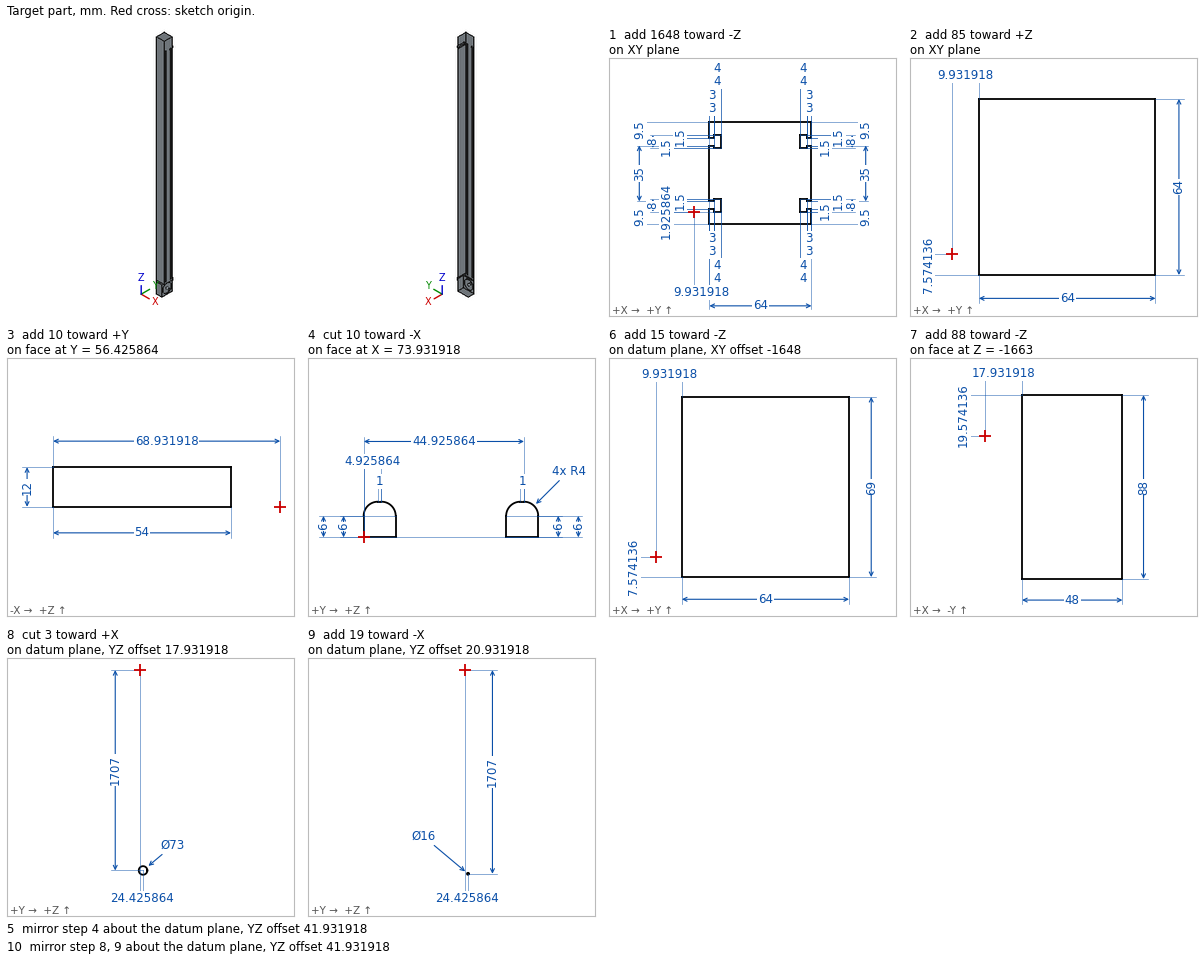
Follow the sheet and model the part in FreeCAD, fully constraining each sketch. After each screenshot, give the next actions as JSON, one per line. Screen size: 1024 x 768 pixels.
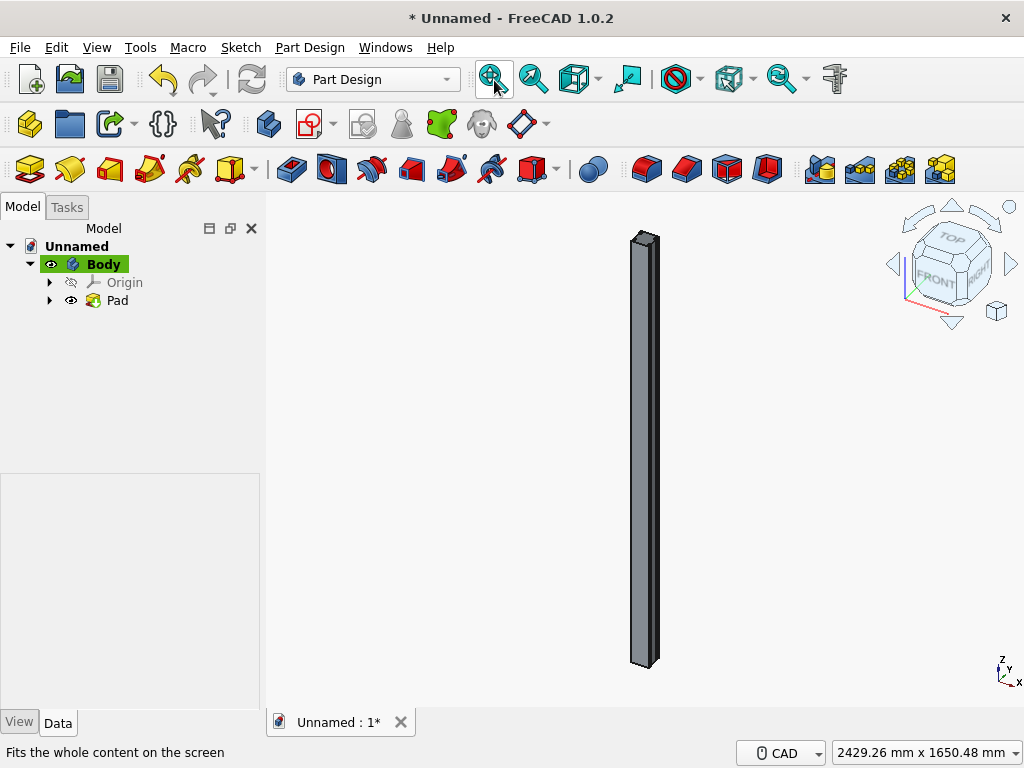
{"action": "left_click", "coordinate": [310, 124]}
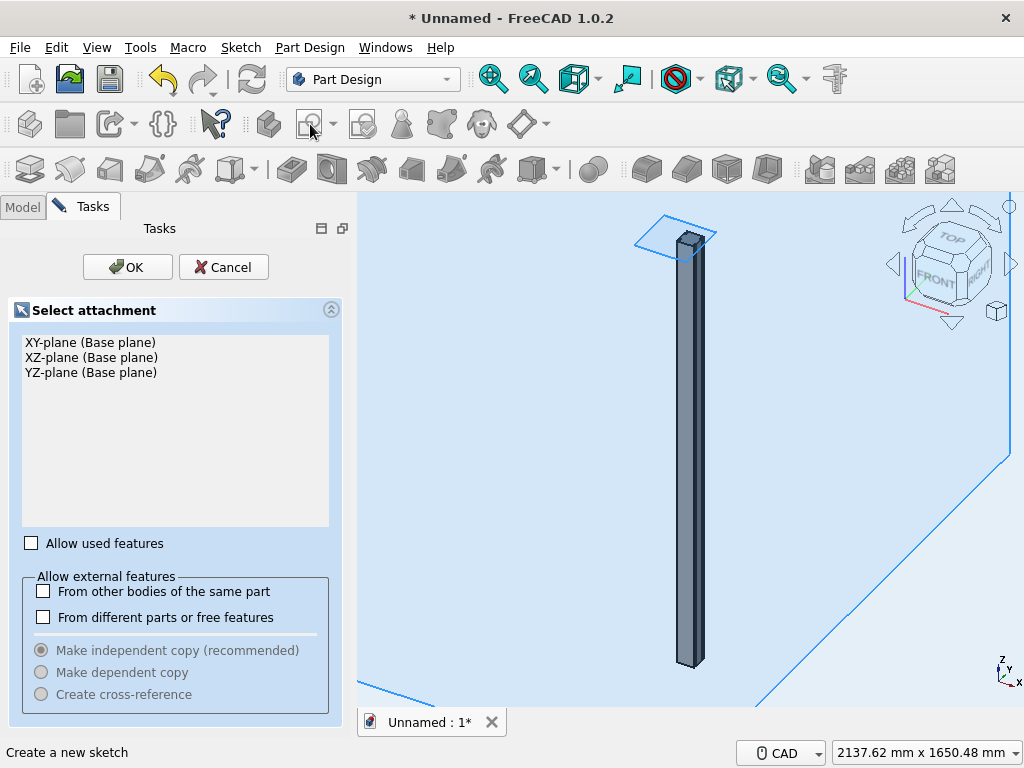
{"action": "left_click", "coordinate": [82, 342]}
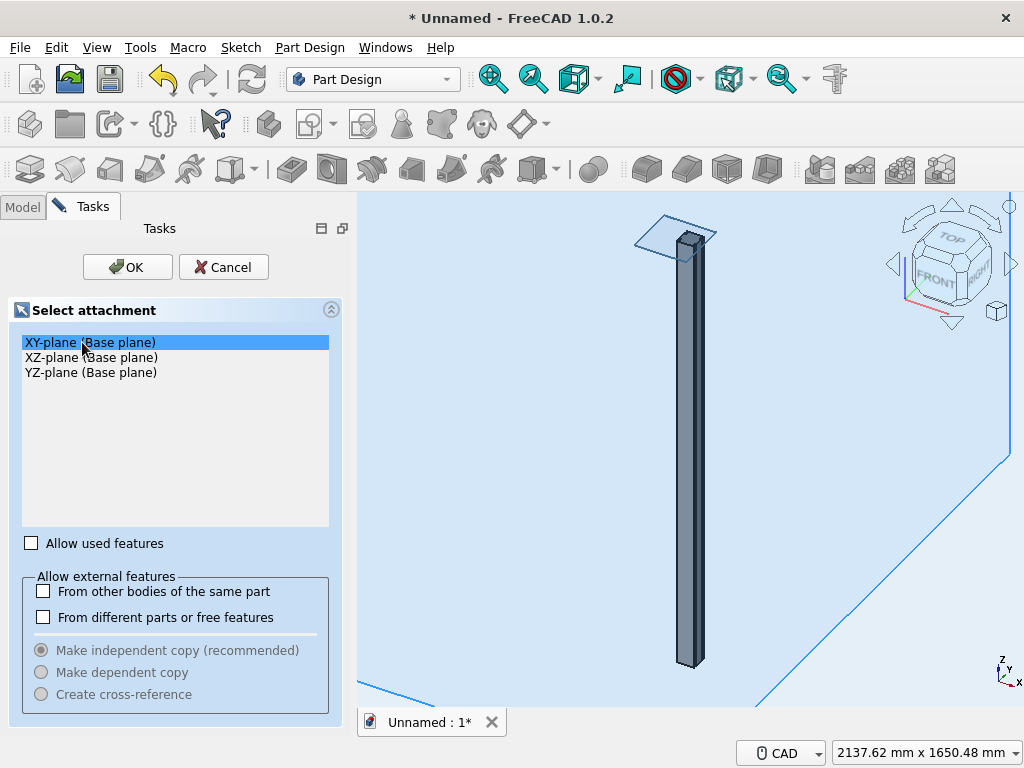
{"action": "left_click", "coordinate": [128, 267]}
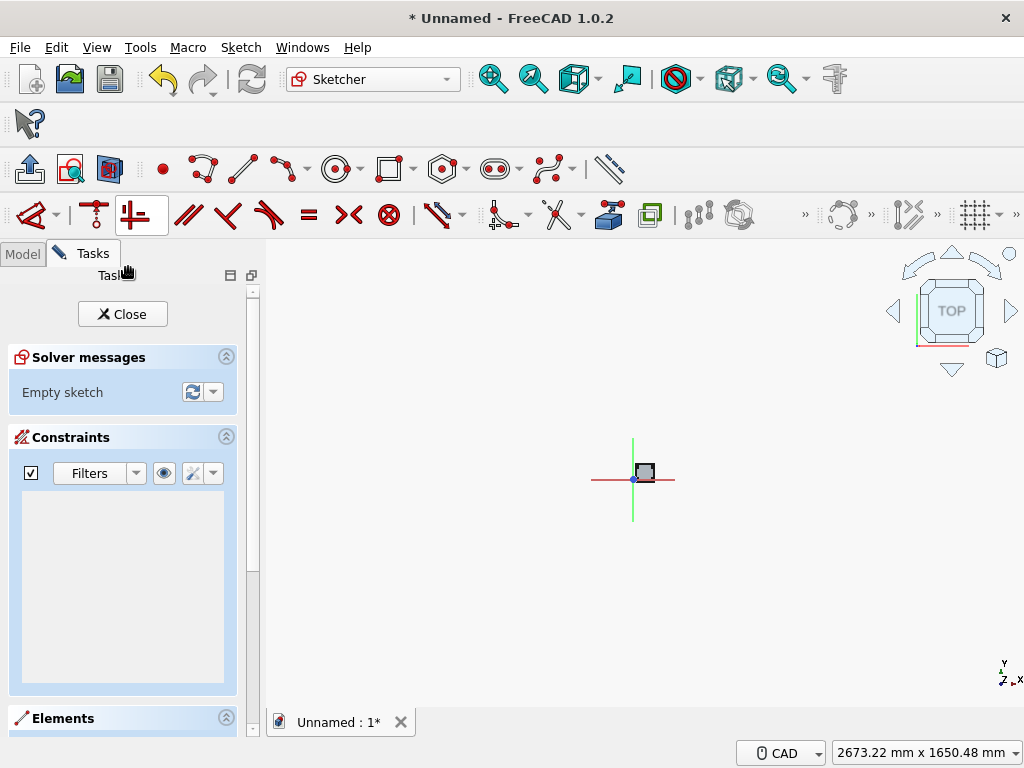
{"action": "scroll", "coordinate": [648, 473], "scroll_direction": "up", "scroll_amount": 14}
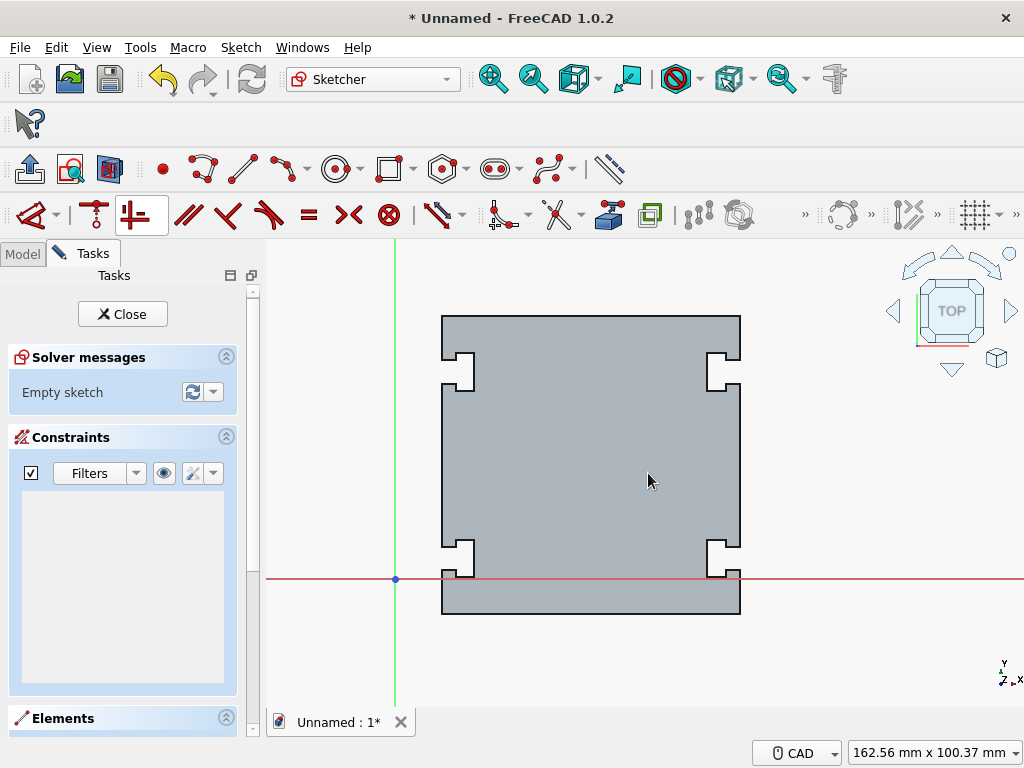
{"action": "left_click", "coordinate": [390, 170]}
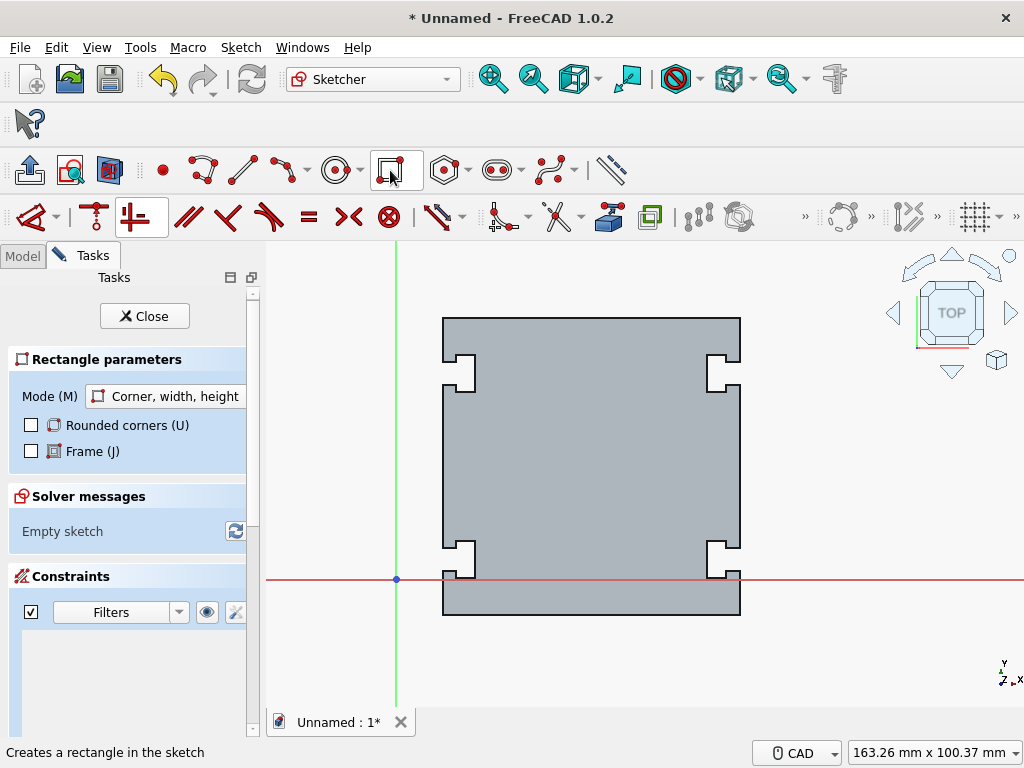
{"action": "left_click", "coordinate": [443, 318]}
{"action": "mouse_move", "coordinate": [740, 615]}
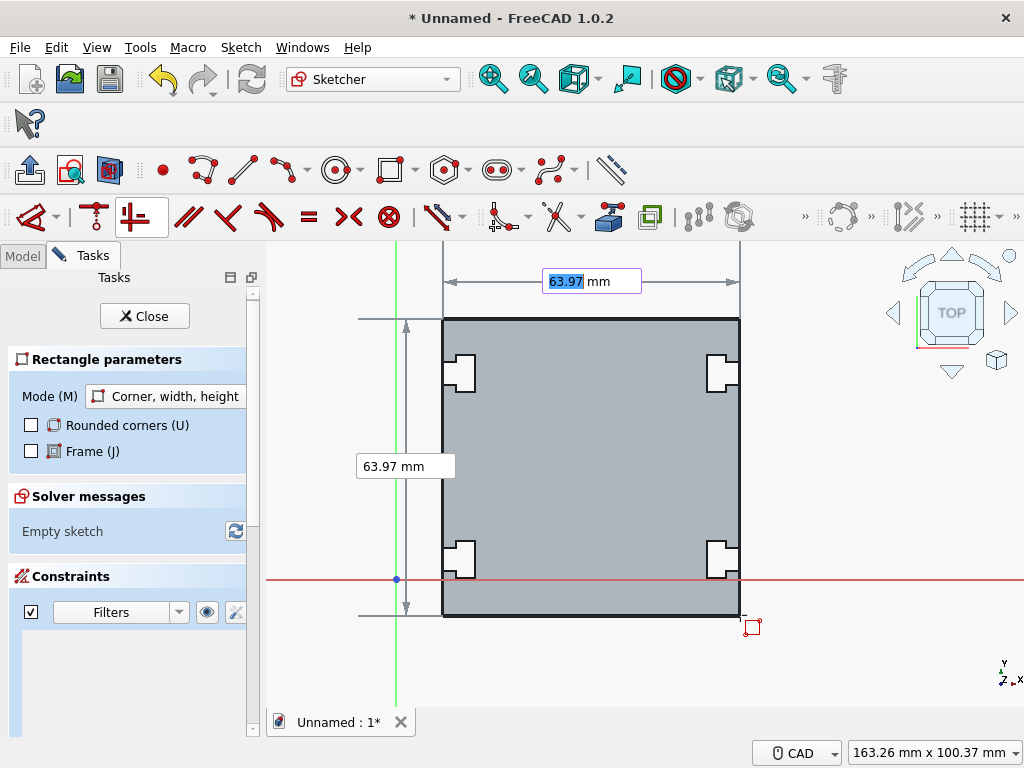
{"action": "type", "text": "64"}
{"action": "key", "text": "Tab"}
{"action": "type", "text": "64"}
{"action": "key", "text": "Return"}
{"action": "key", "text": "Escape"}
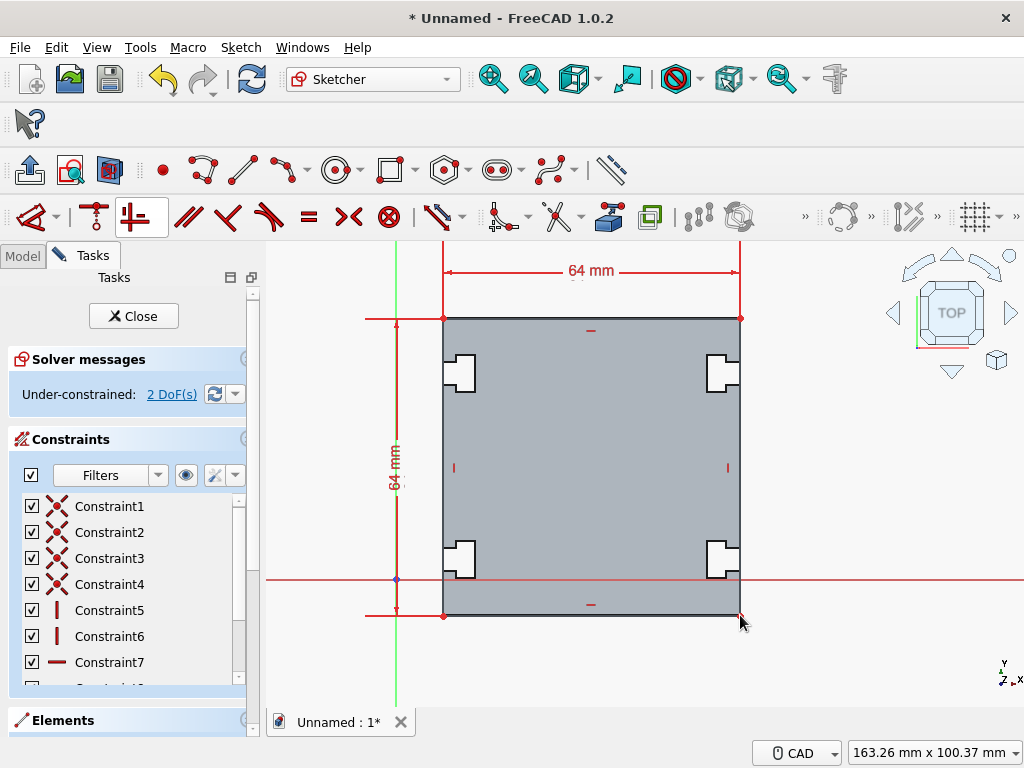
{"action": "left_click", "coordinate": [32, 218]}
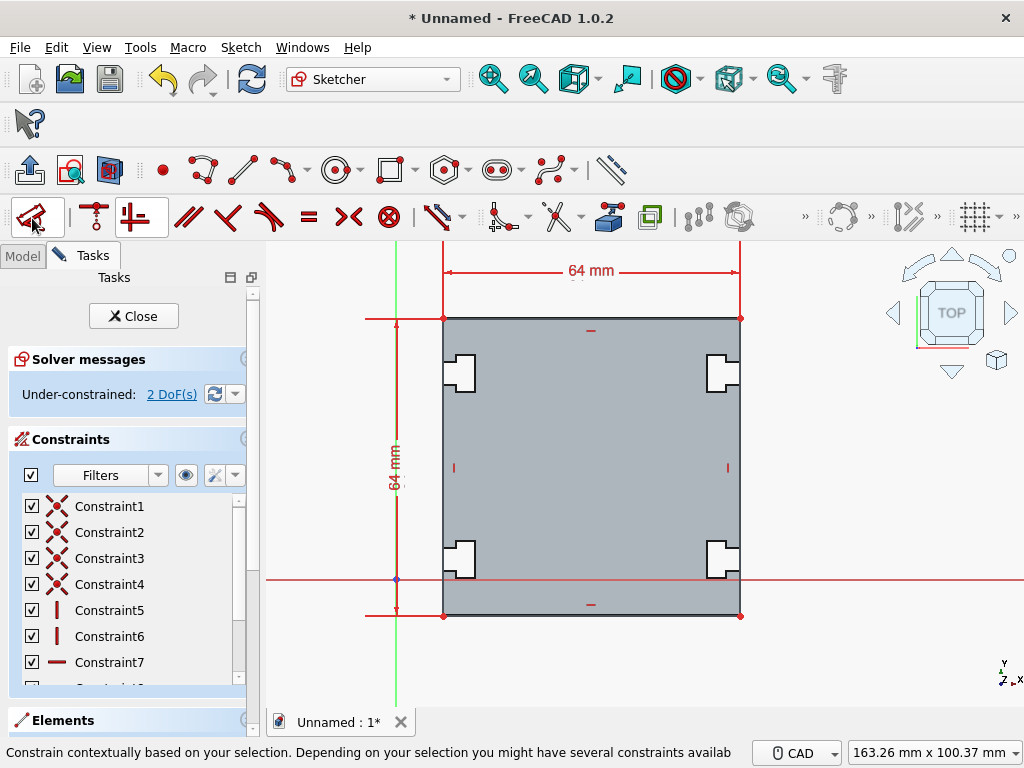
{"action": "left_click", "coordinate": [443, 319]}
{"action": "left_click", "coordinate": [420, 285]}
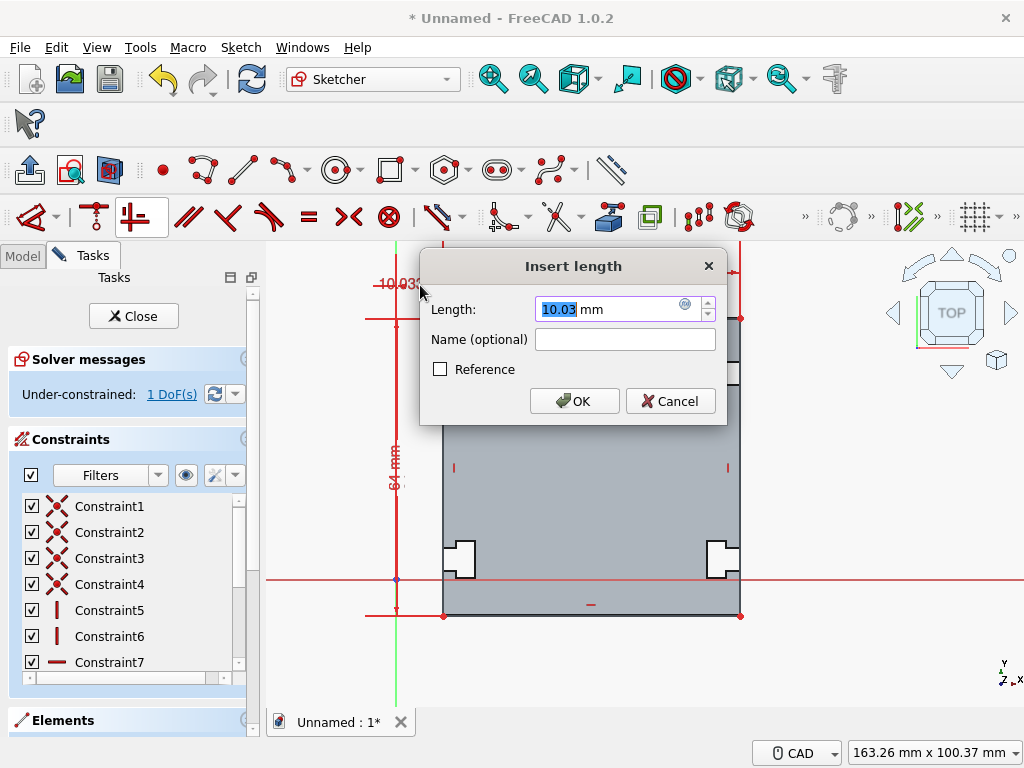
{"action": "type", "text": "9.931918"}
{"action": "key", "text": "Return"}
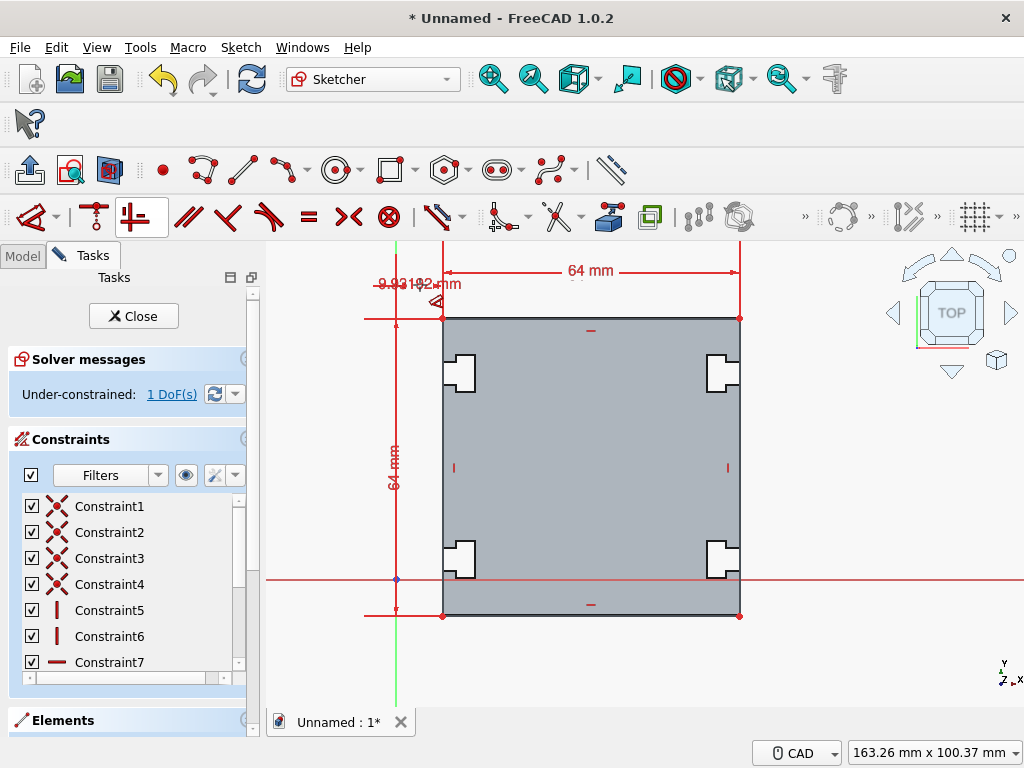
{"action": "left_click", "coordinate": [443, 616]}
{"action": "left_click", "coordinate": [362, 598]}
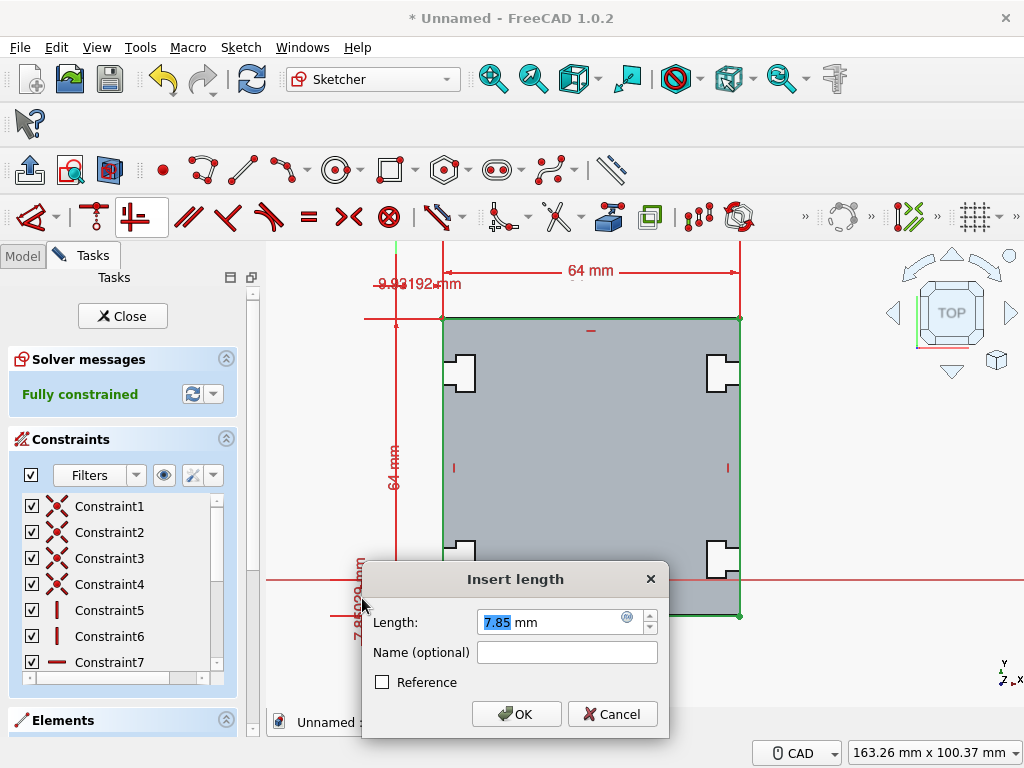
{"action": "type", "text": "7.574136"}
{"action": "key", "text": "Return"}
{"action": "key", "text": "Escape"}